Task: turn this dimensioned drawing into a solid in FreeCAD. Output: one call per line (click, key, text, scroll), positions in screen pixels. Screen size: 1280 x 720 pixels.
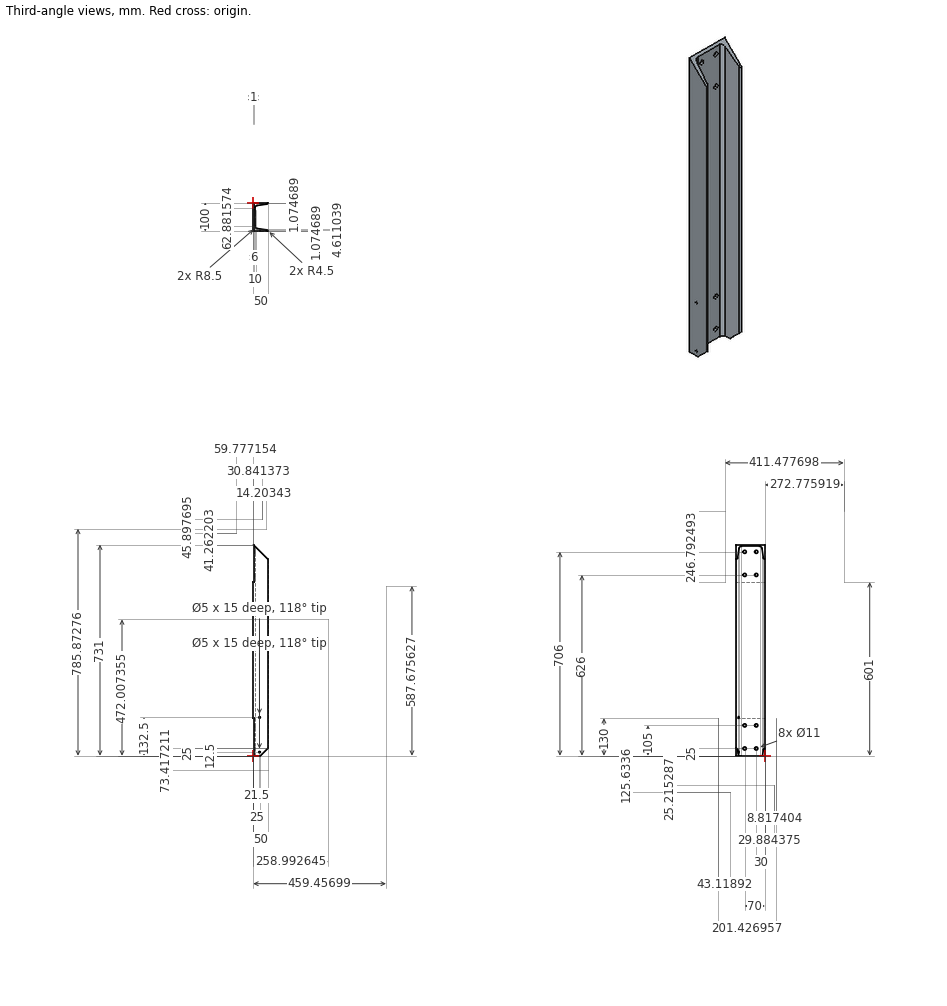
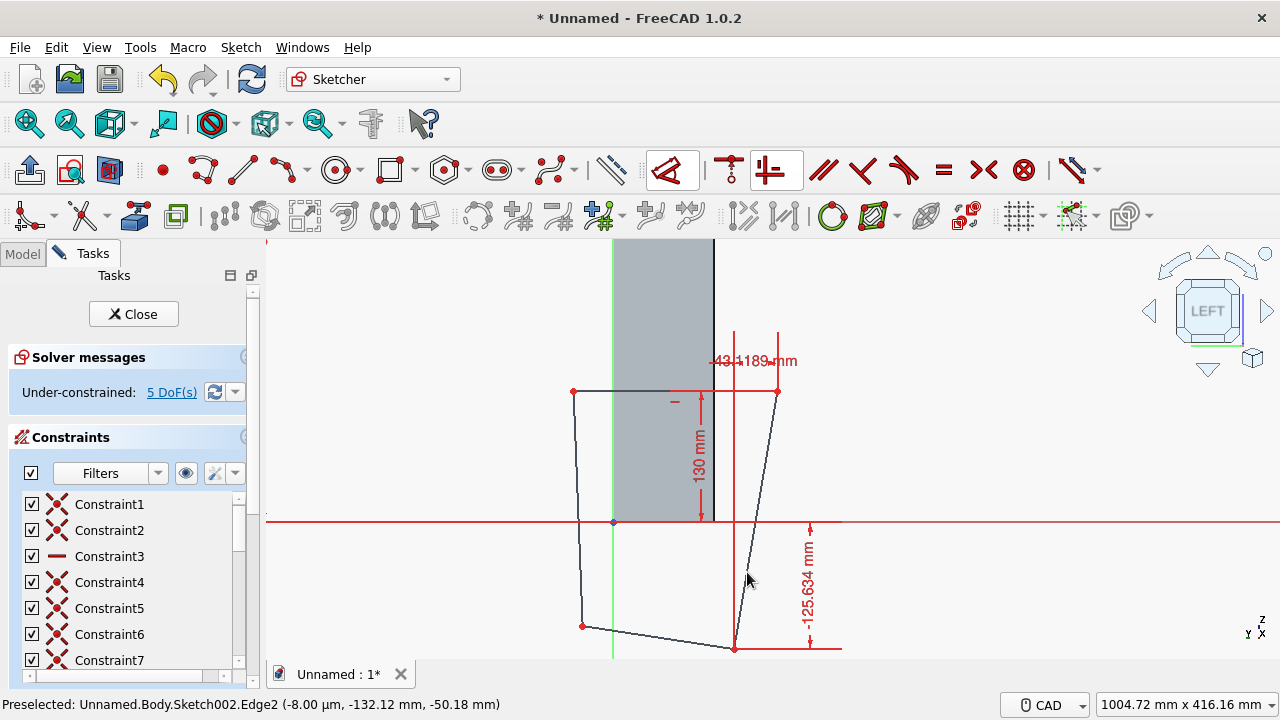
scroll(576, 462, up, 8)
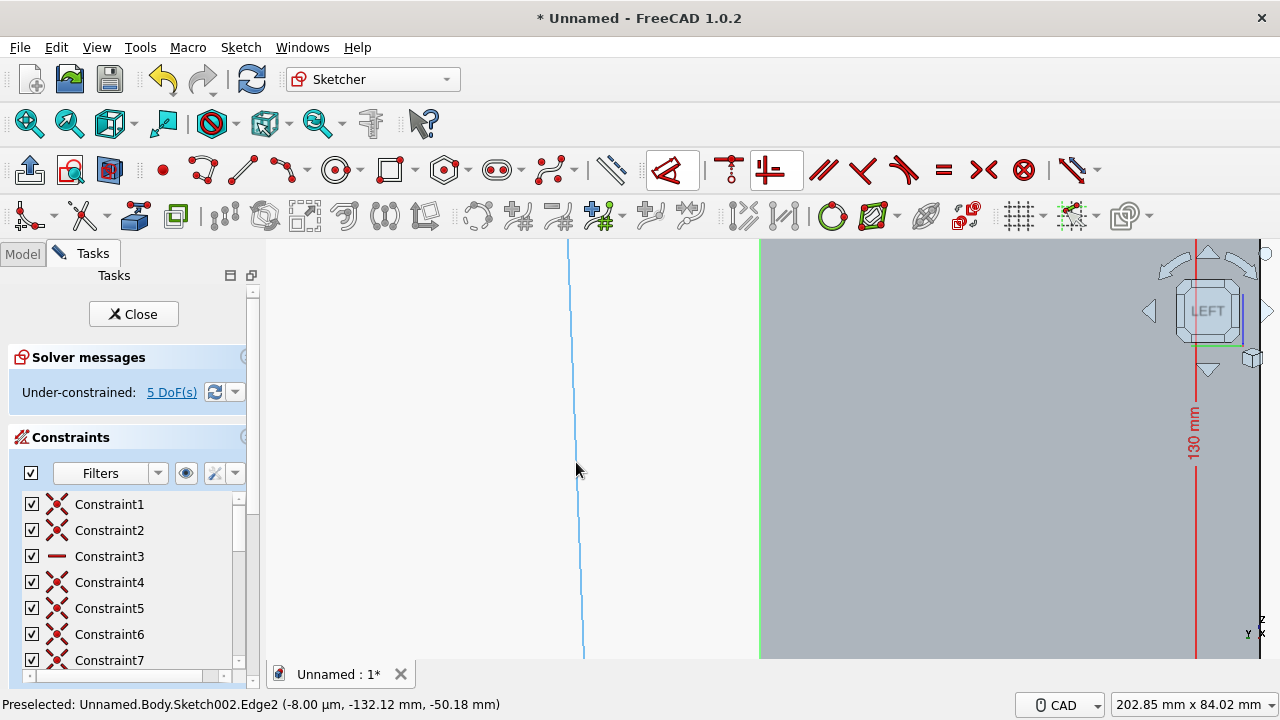
click(576, 458)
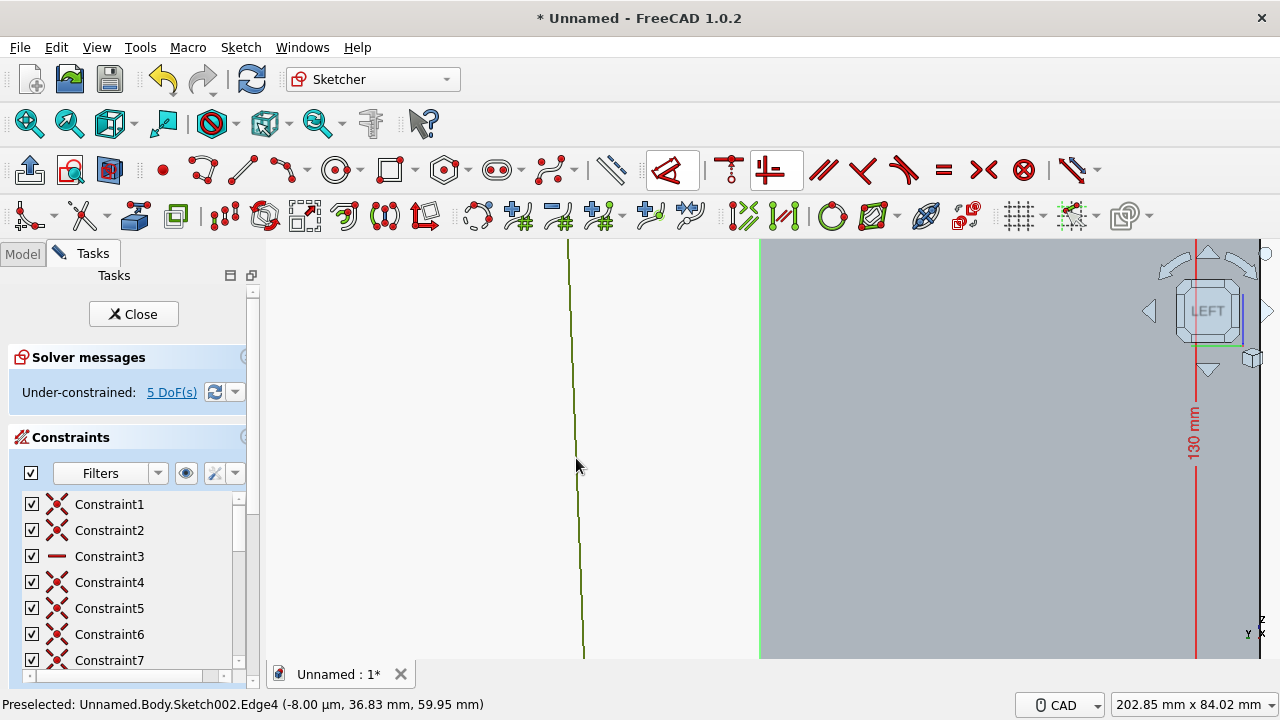
key(l)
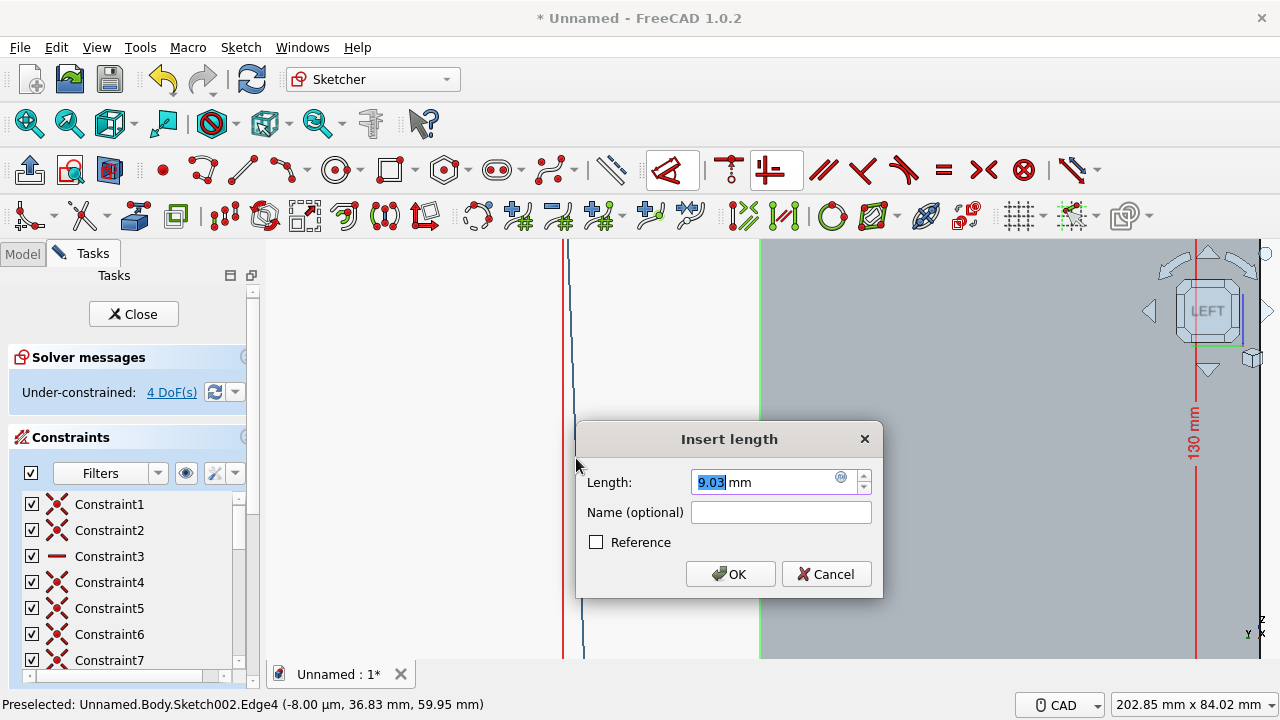
text(8.817404)
key(Return)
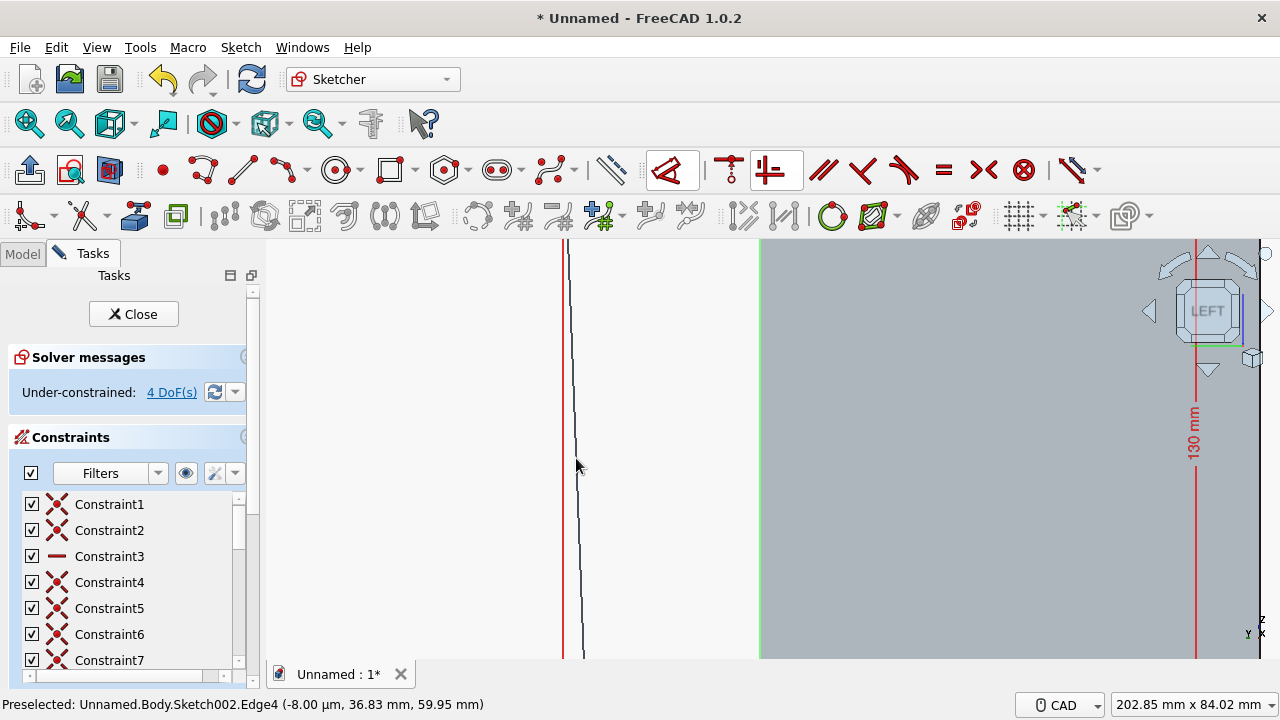
scroll(716, 527, down, 15)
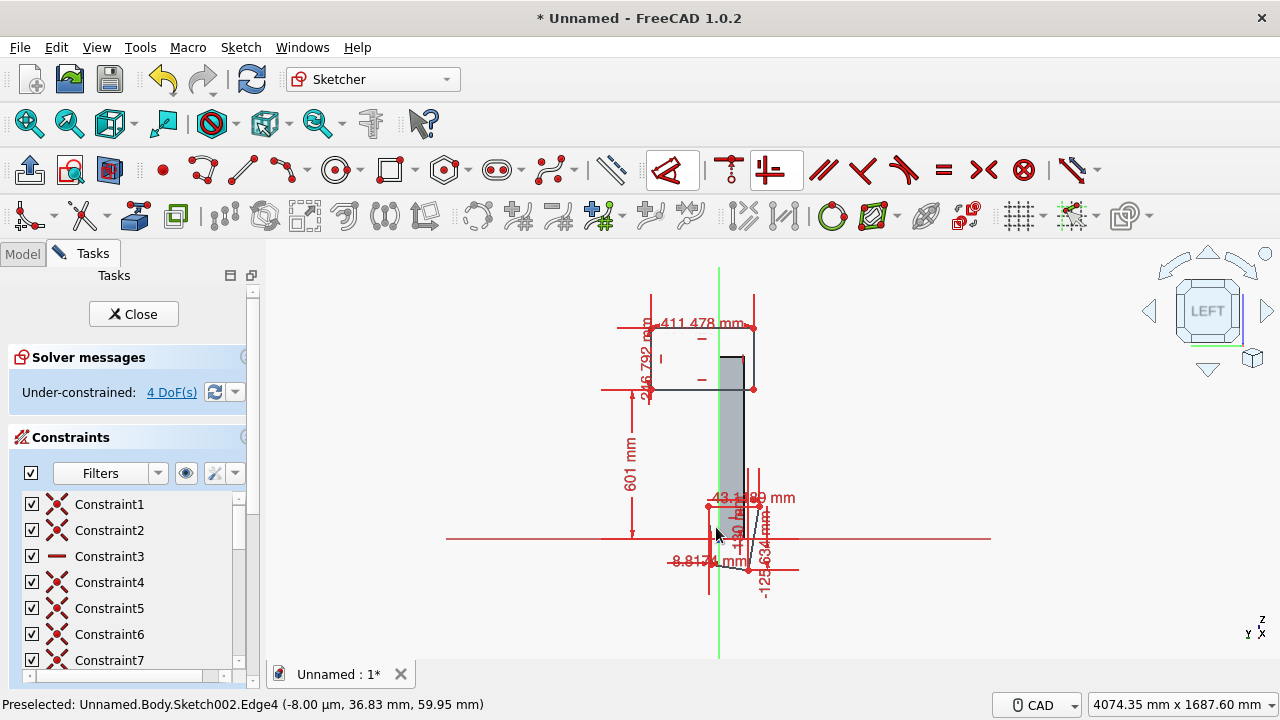
click(724, 507)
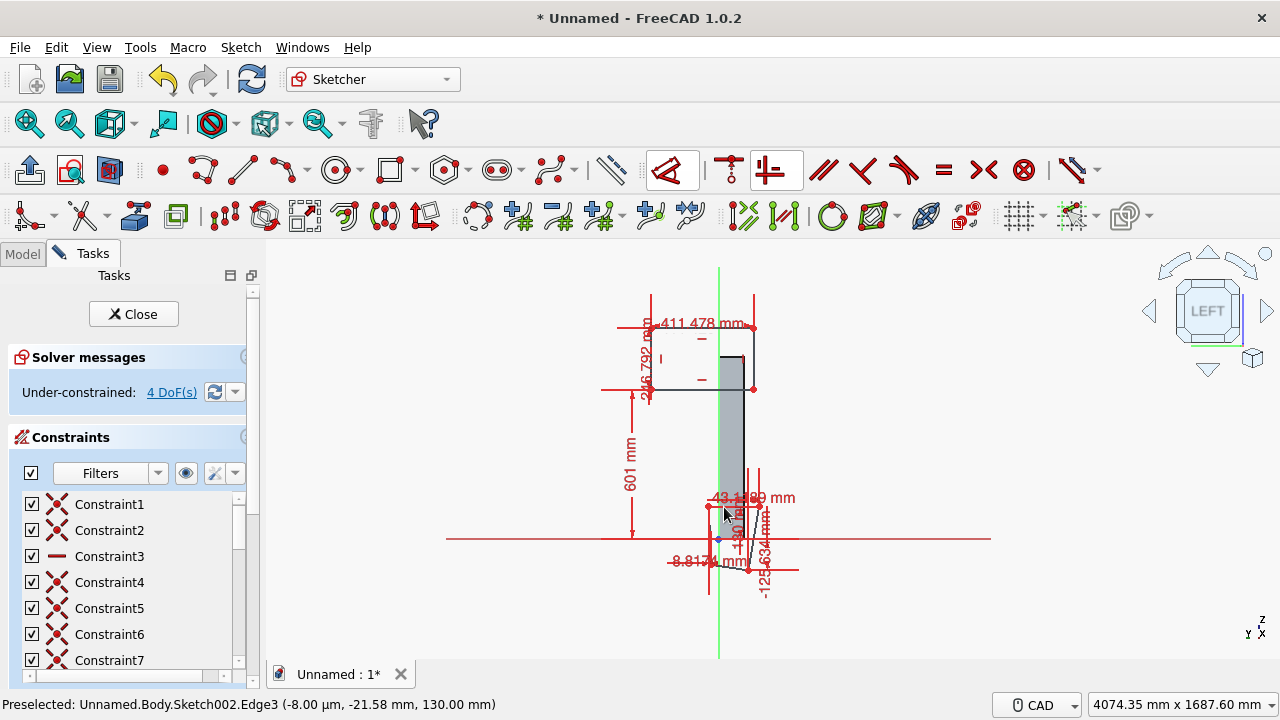
key(l)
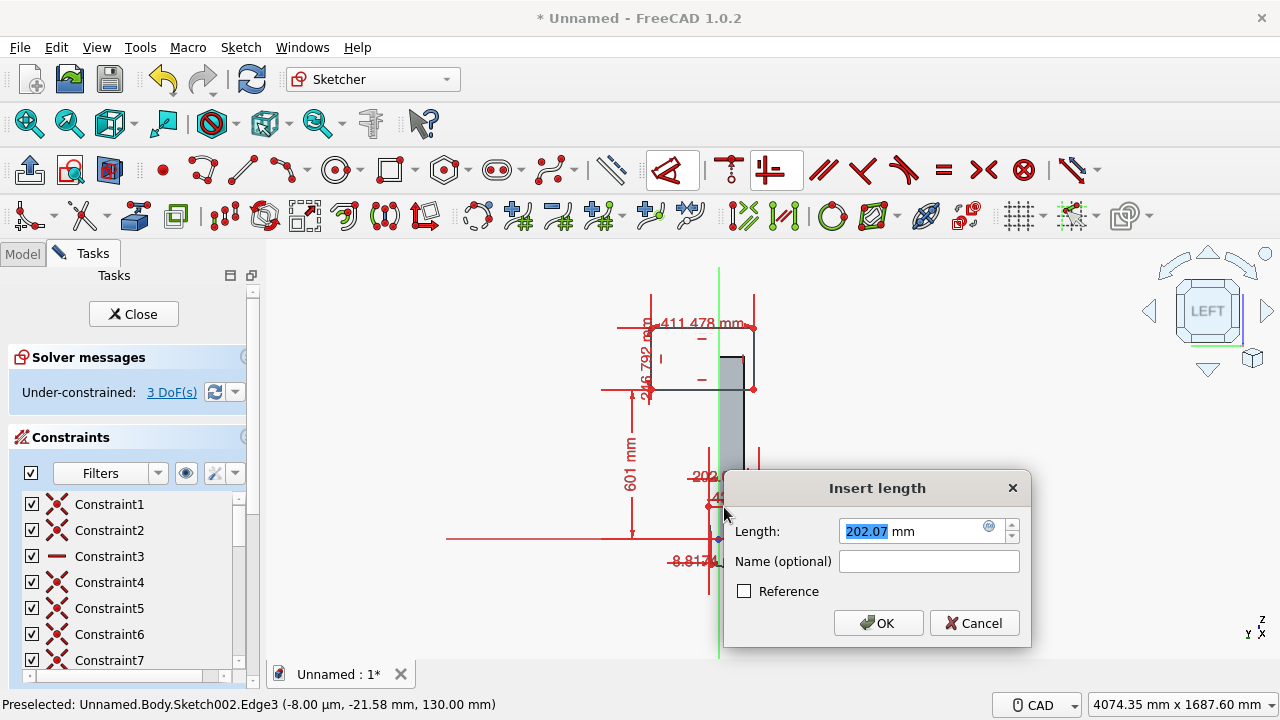
text(201.426957)
key(Return)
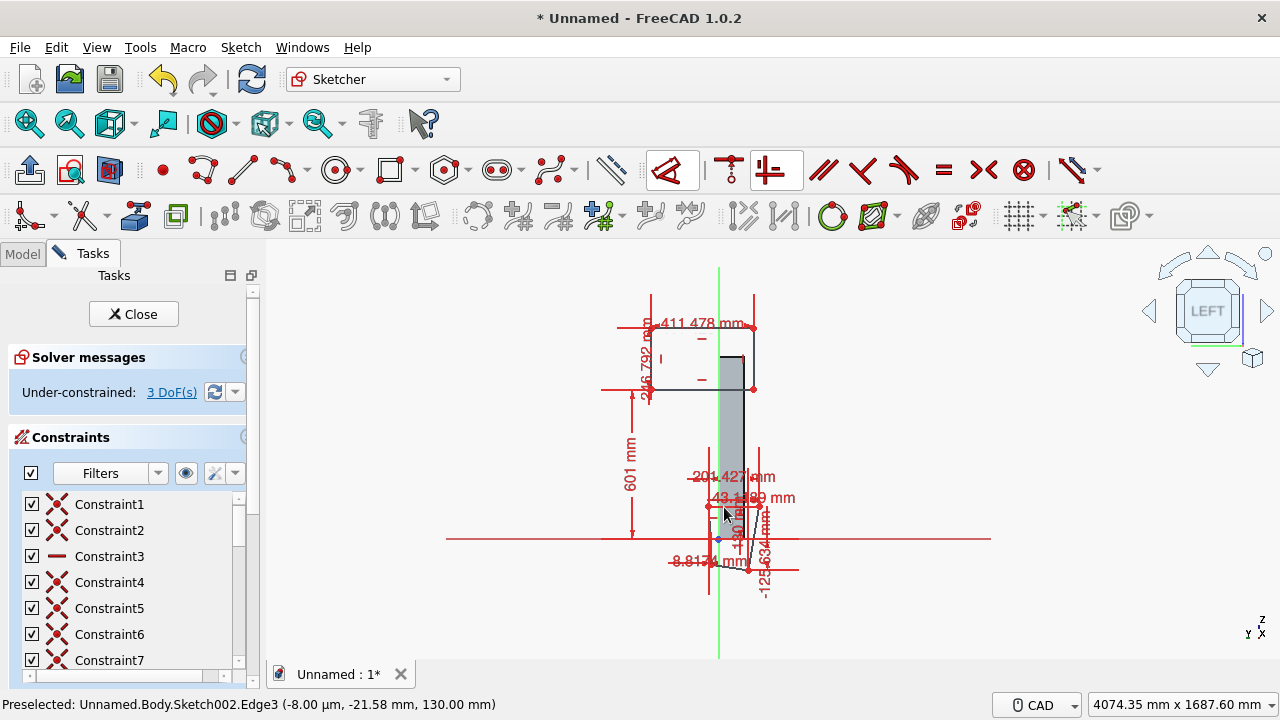
scroll(711, 565, up, 9)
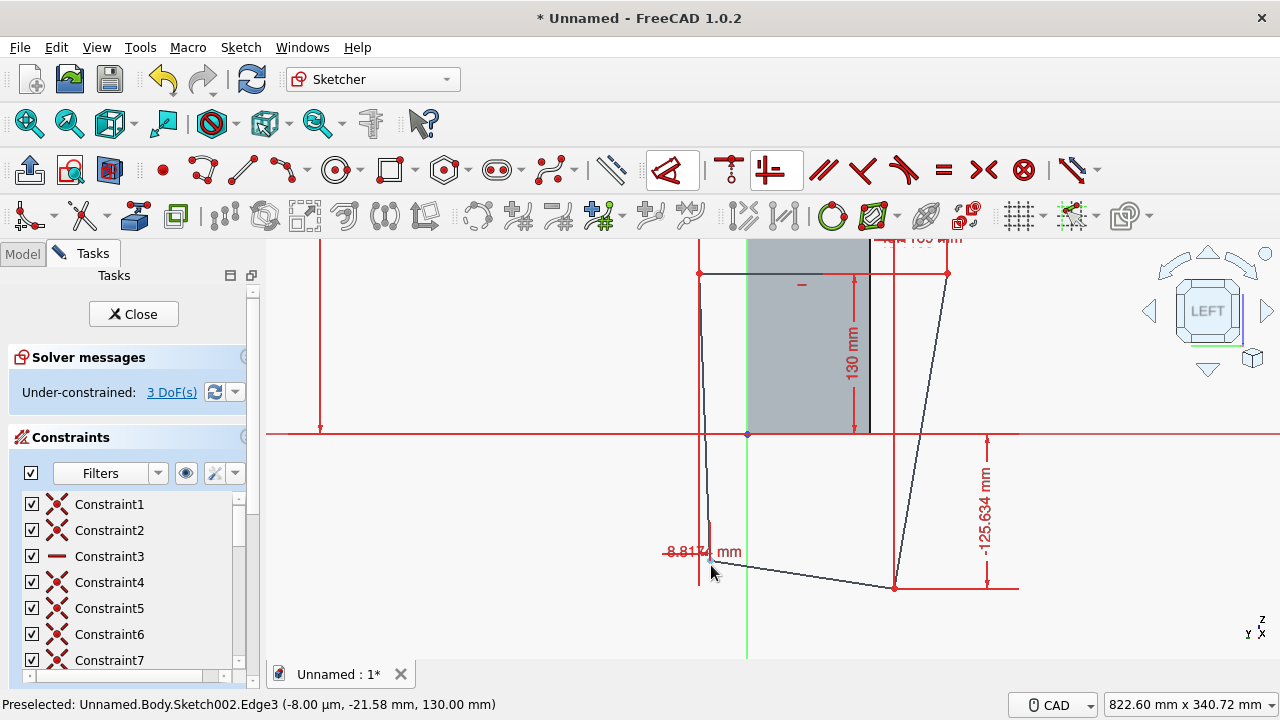
click(710, 560)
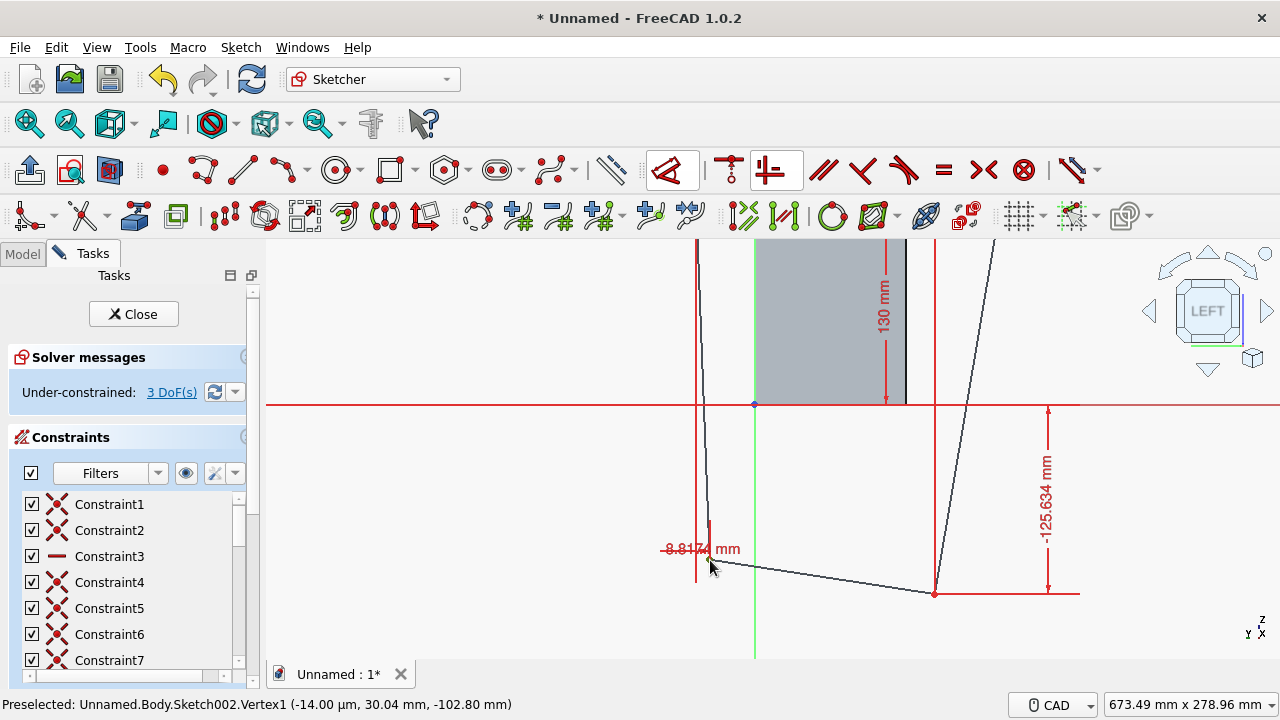
key(l)